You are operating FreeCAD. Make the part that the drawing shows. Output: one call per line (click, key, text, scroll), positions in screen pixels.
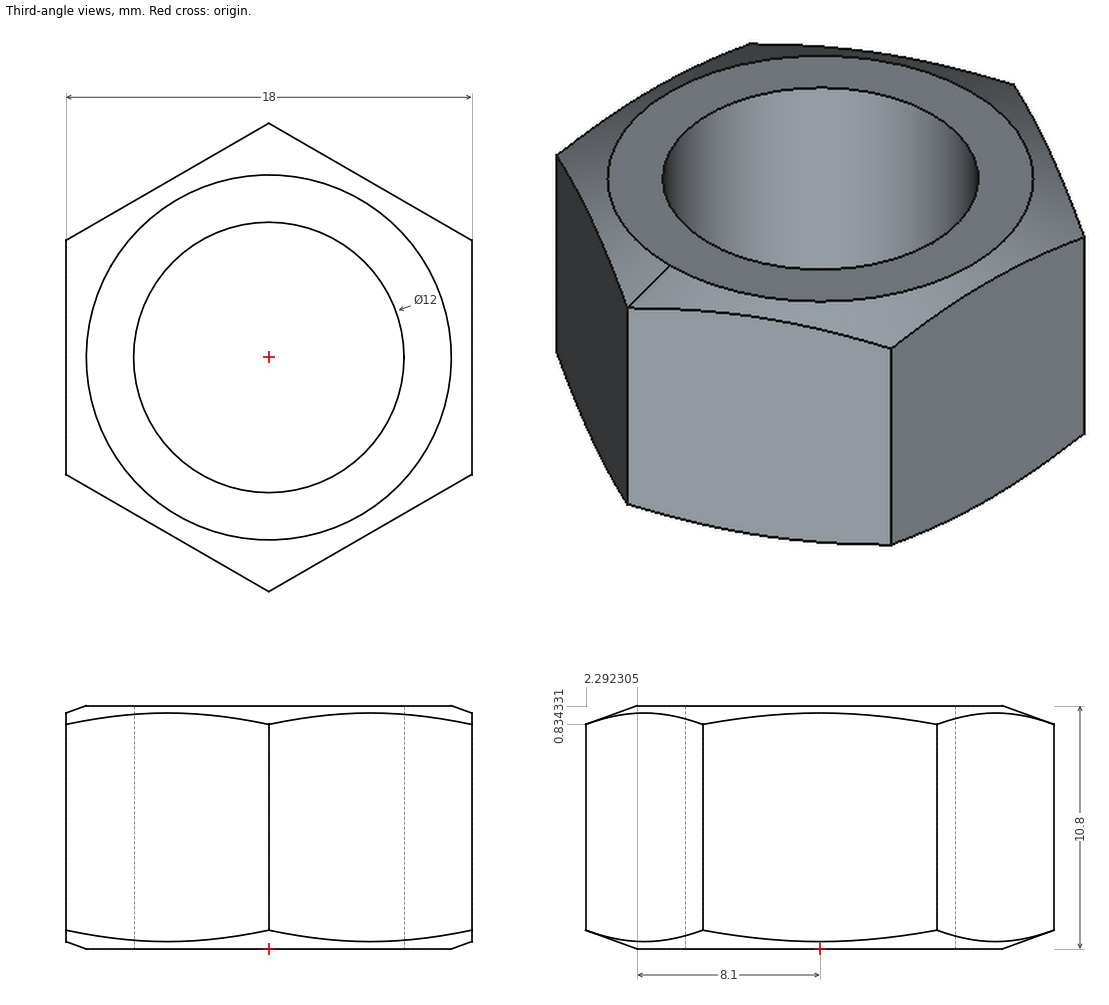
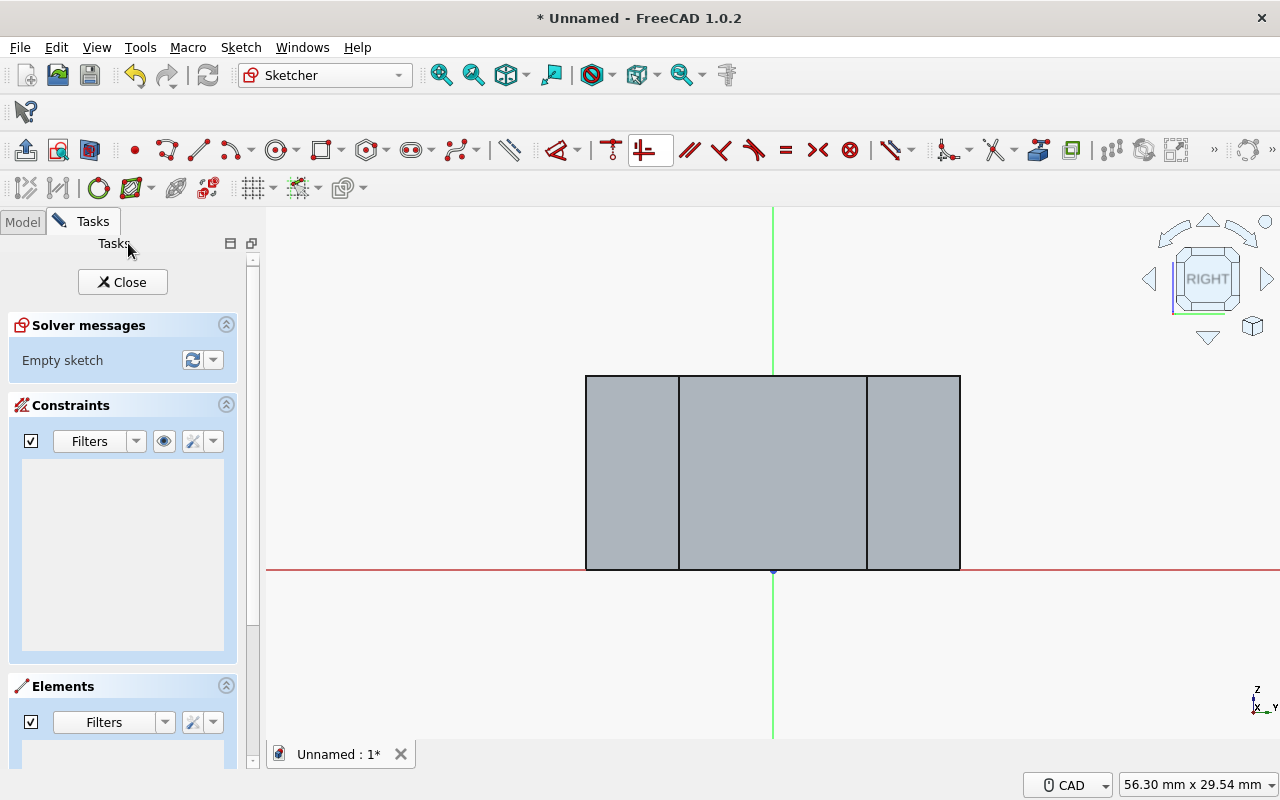
click(90, 150)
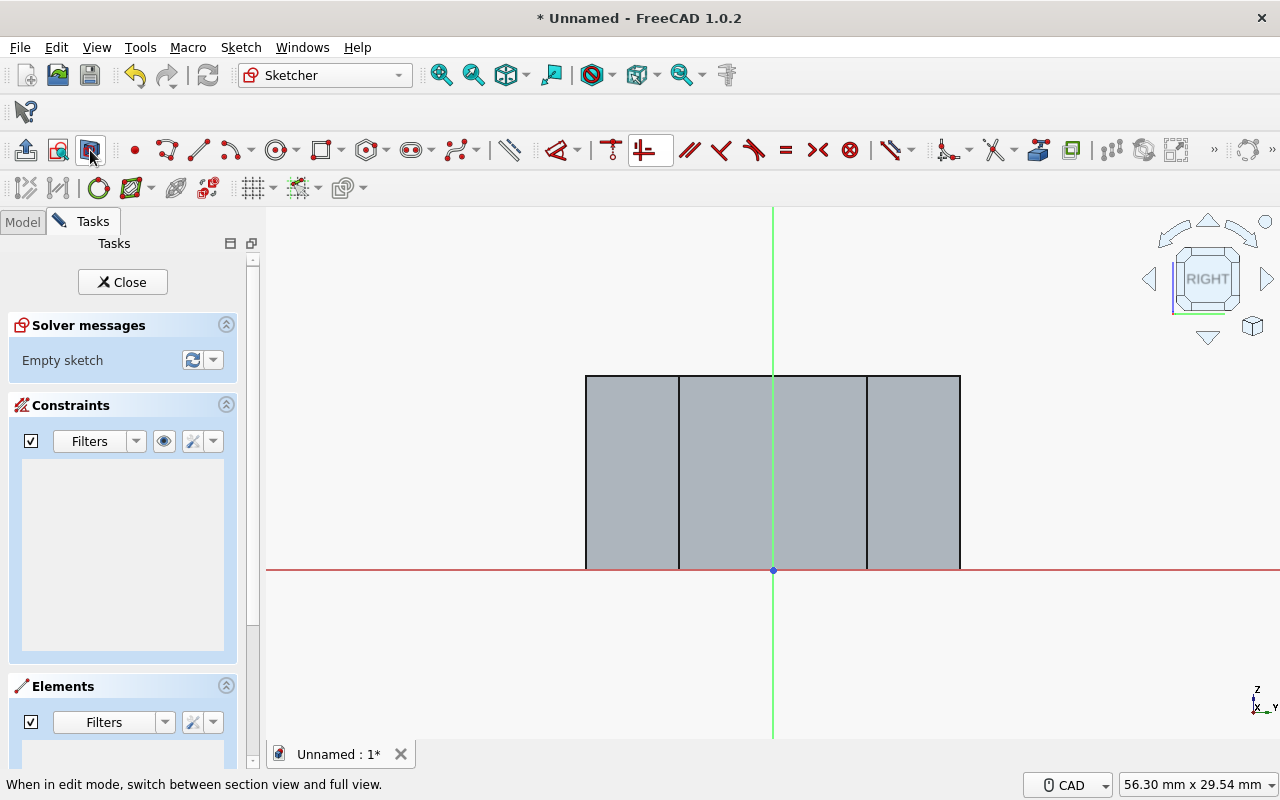
scroll(599, 376, up, 13)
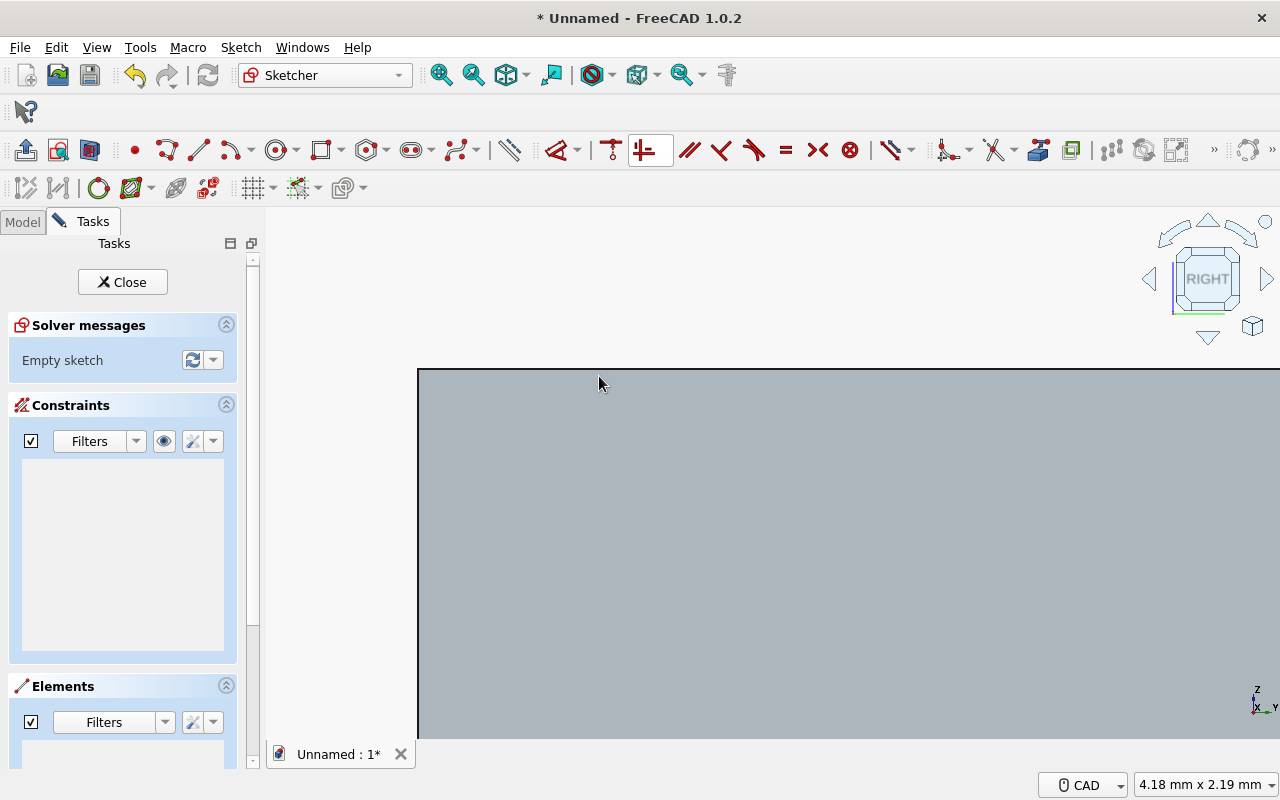
click(168, 150)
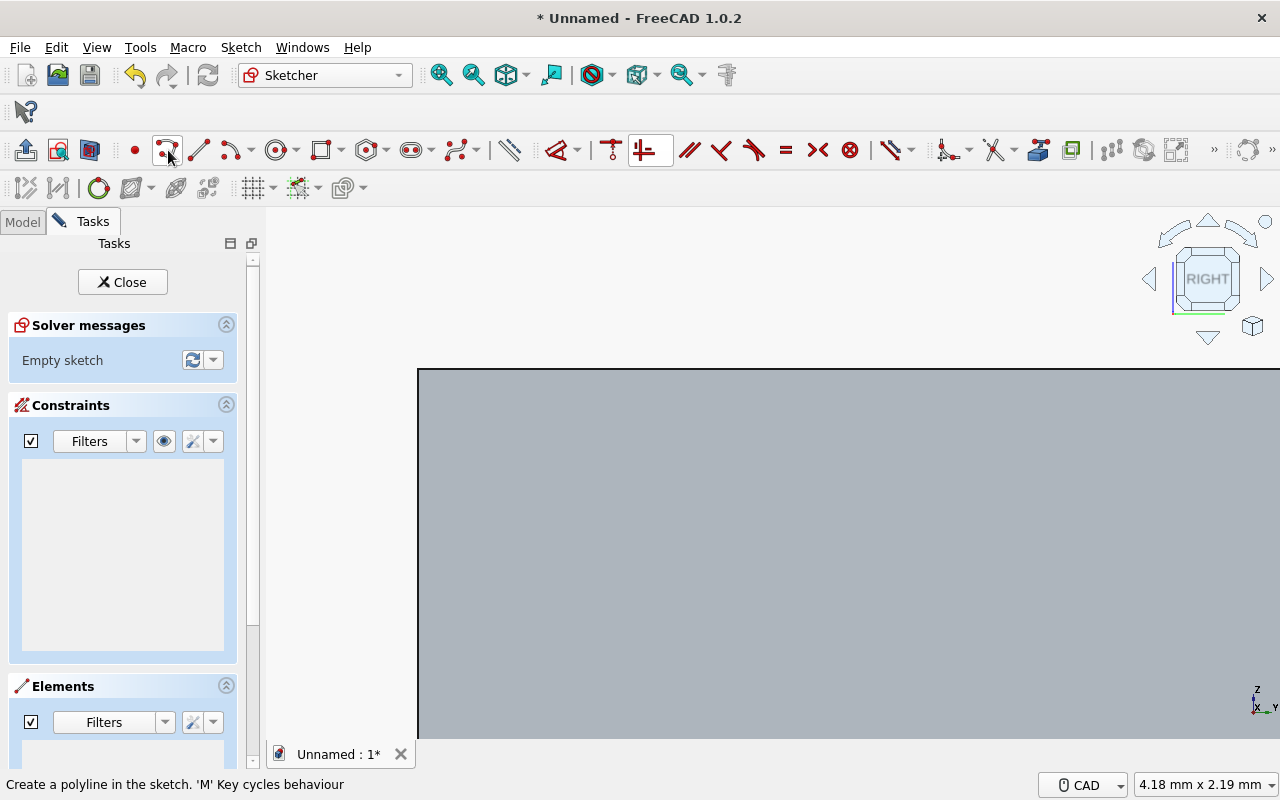
click(974, 369)
click(418, 369)
click(418, 571)
click(974, 370)
key(Escape)
key(Escape)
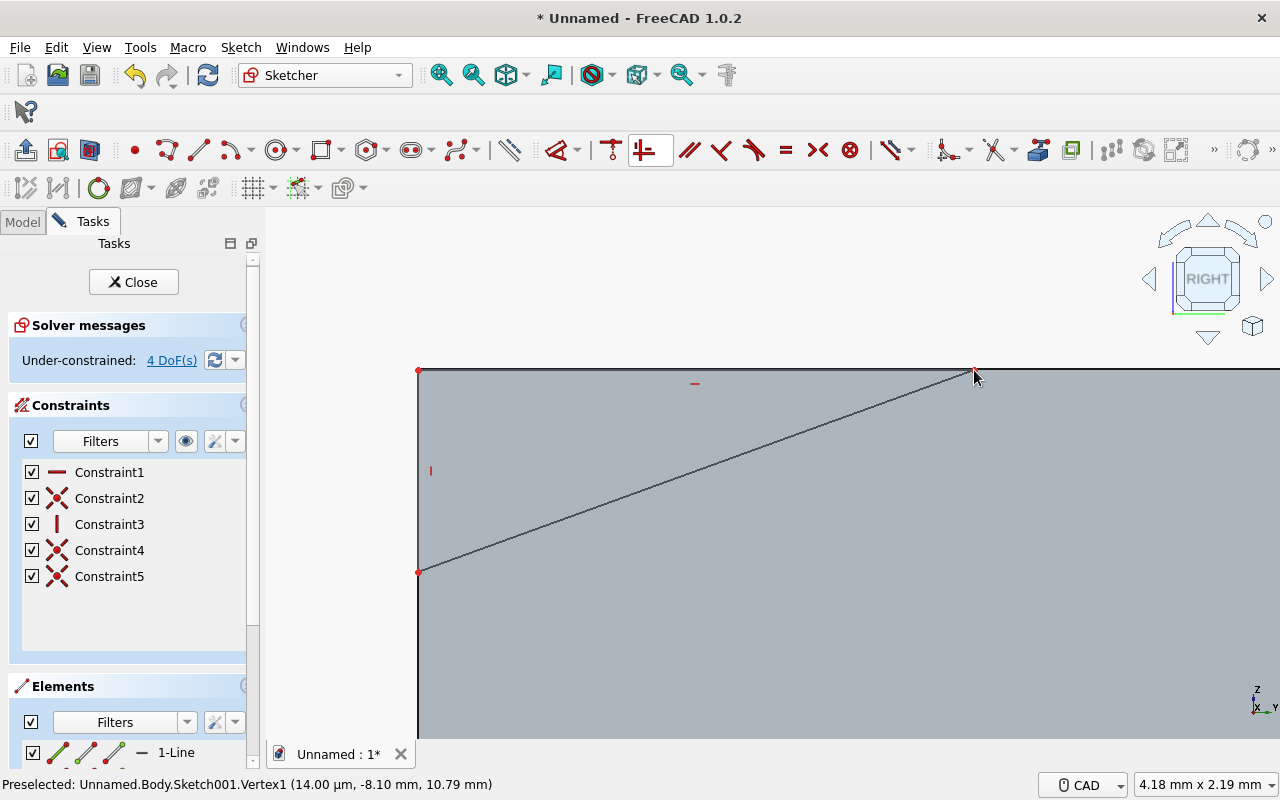
click(556, 150)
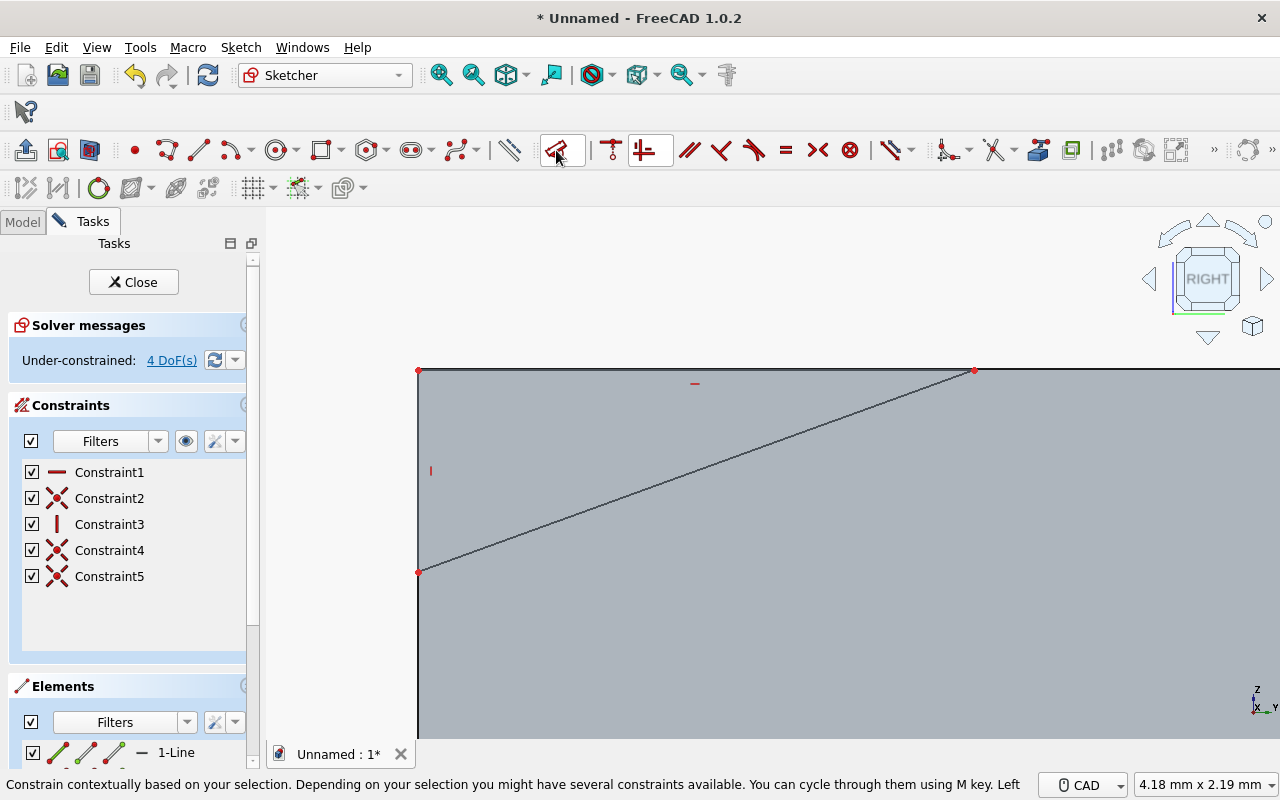
click(974, 370)
click(1044, 336)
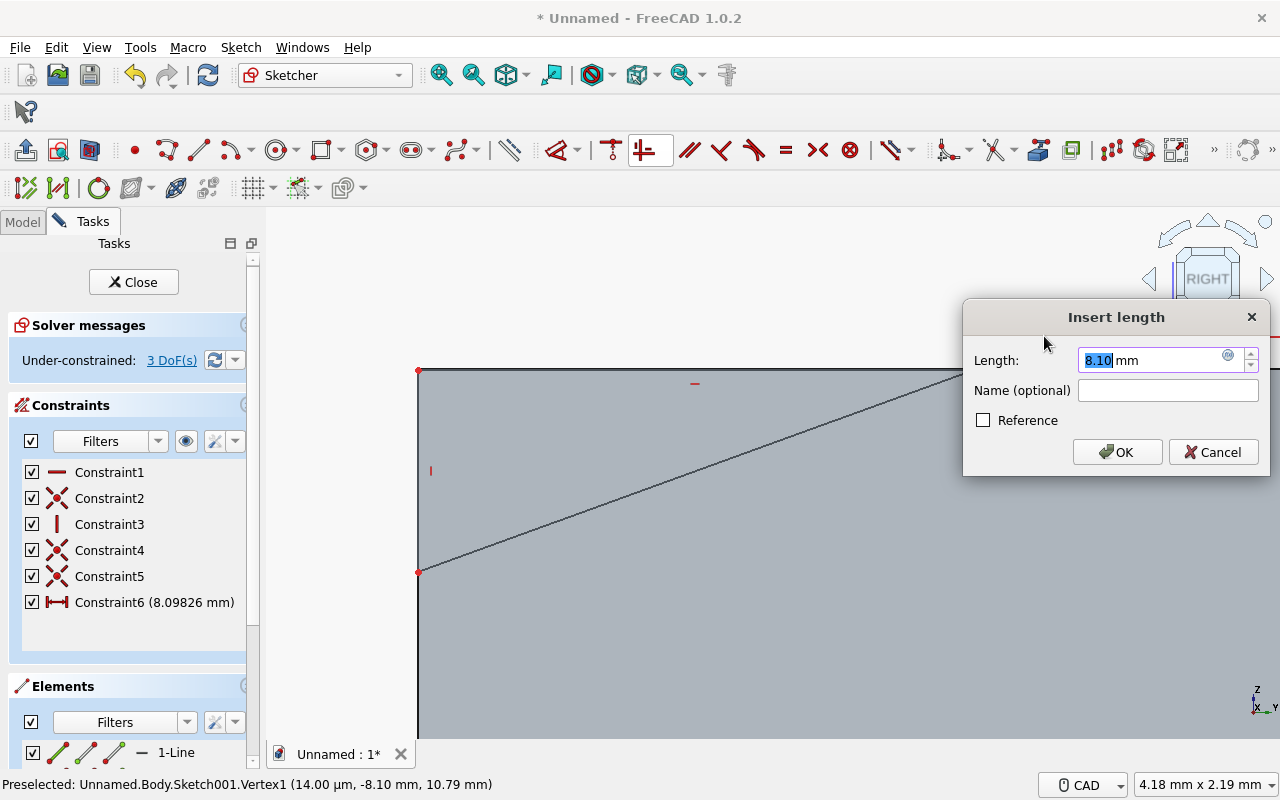
text(8.1)
key(Return)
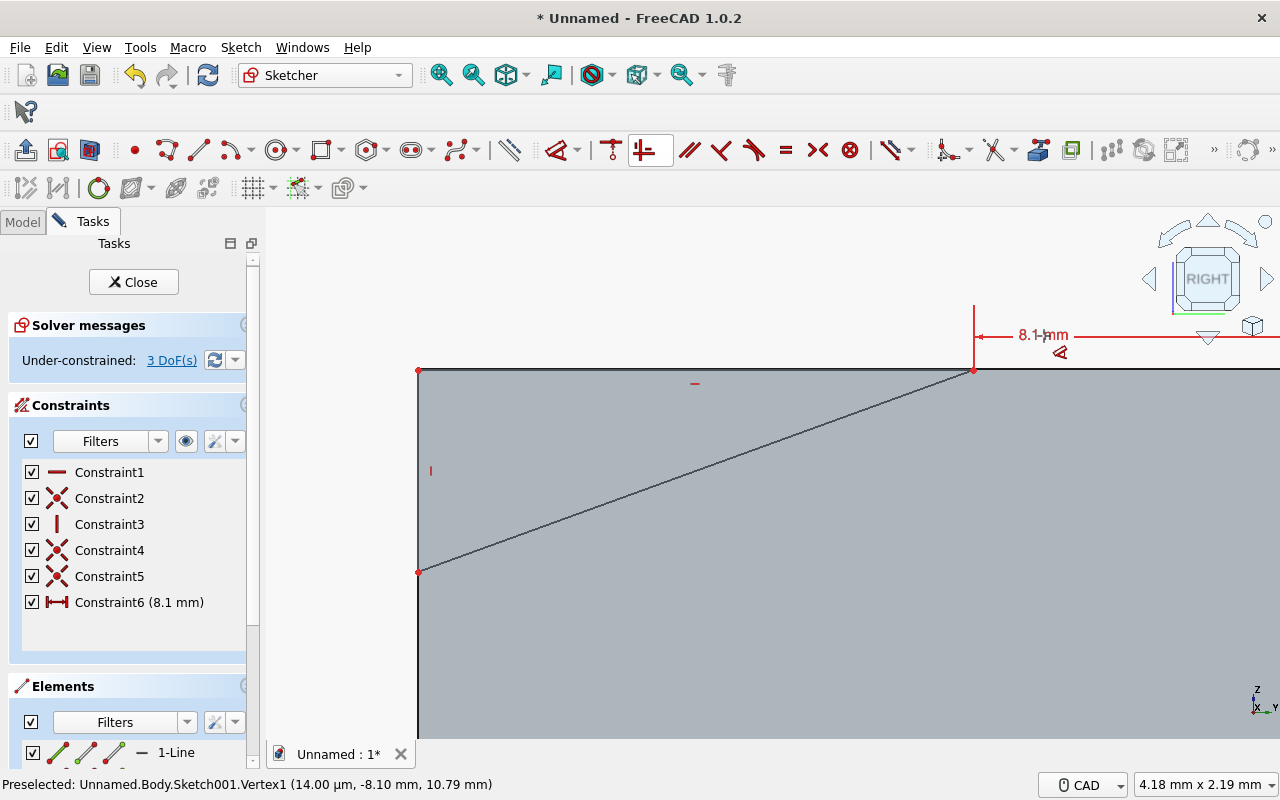
click(974, 370)
click(940, 541)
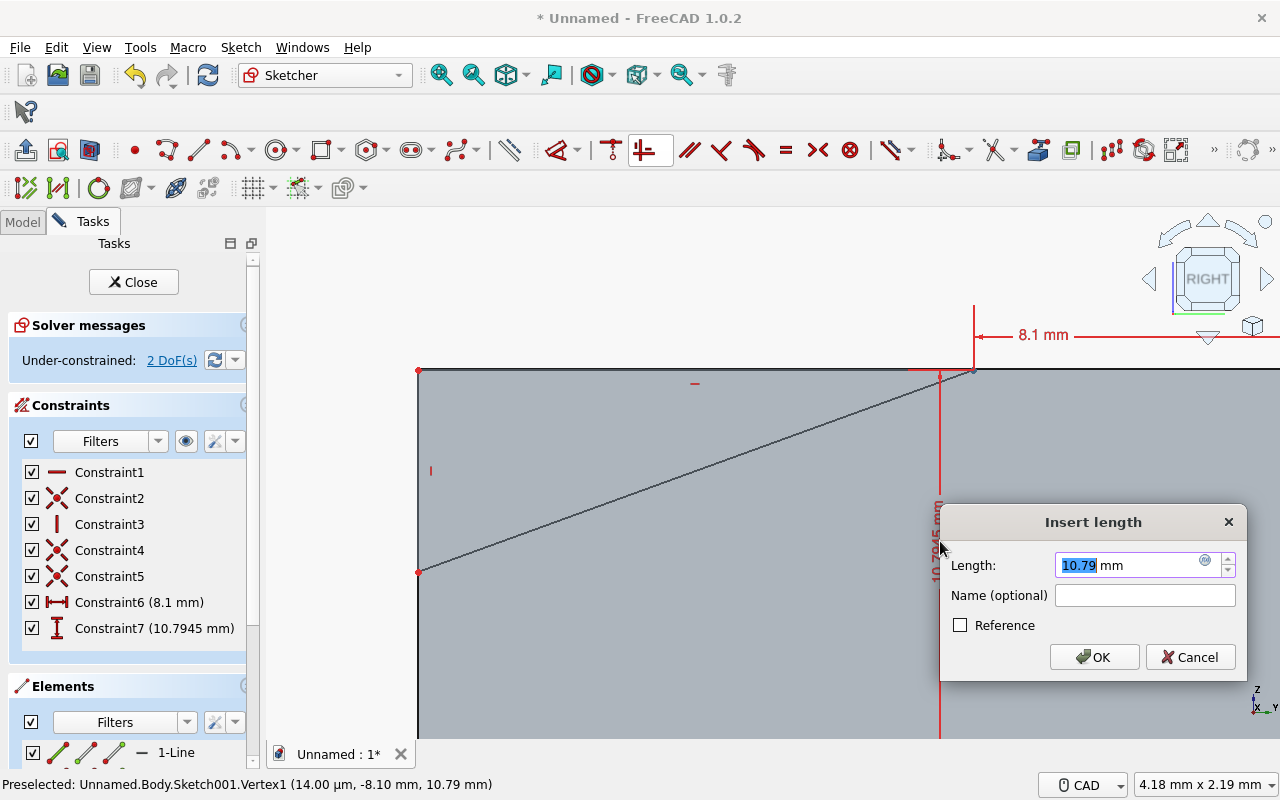
text(10.8)
key(Return)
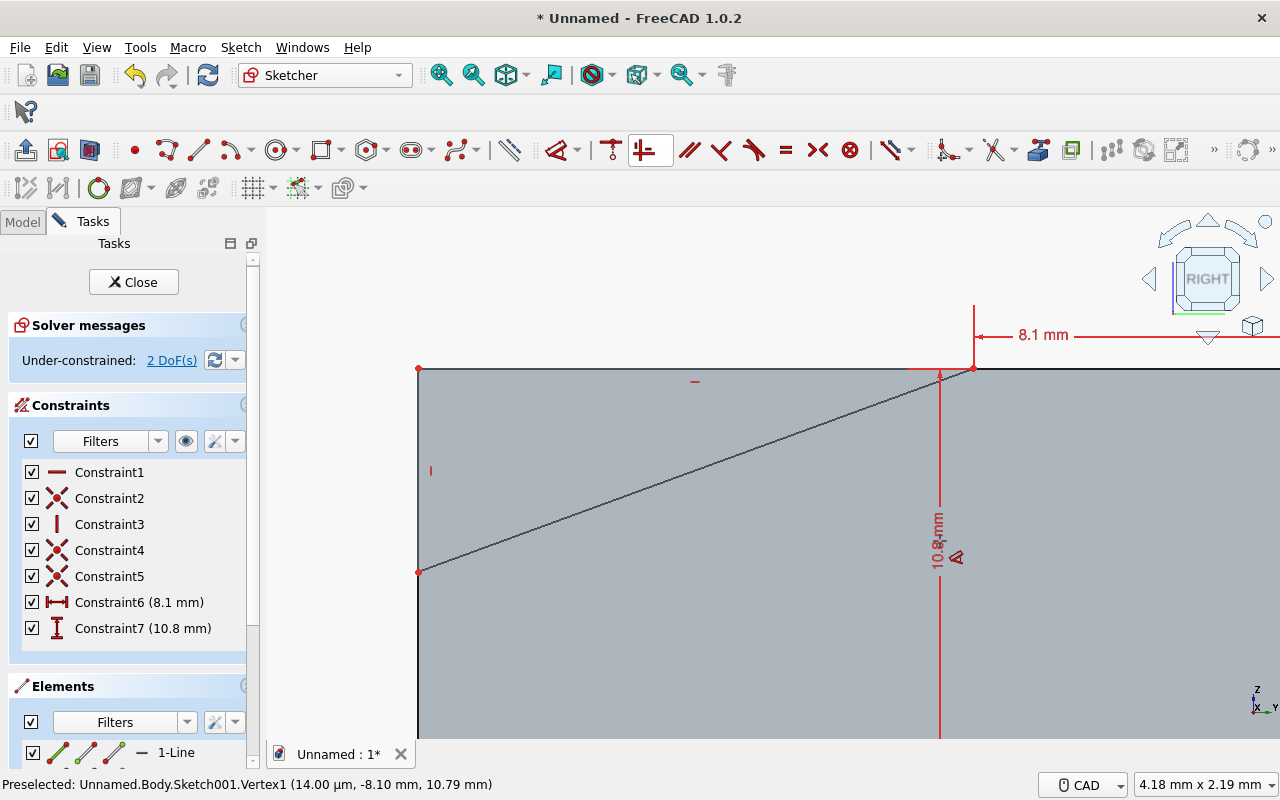
click(807, 369)
click(696, 335)